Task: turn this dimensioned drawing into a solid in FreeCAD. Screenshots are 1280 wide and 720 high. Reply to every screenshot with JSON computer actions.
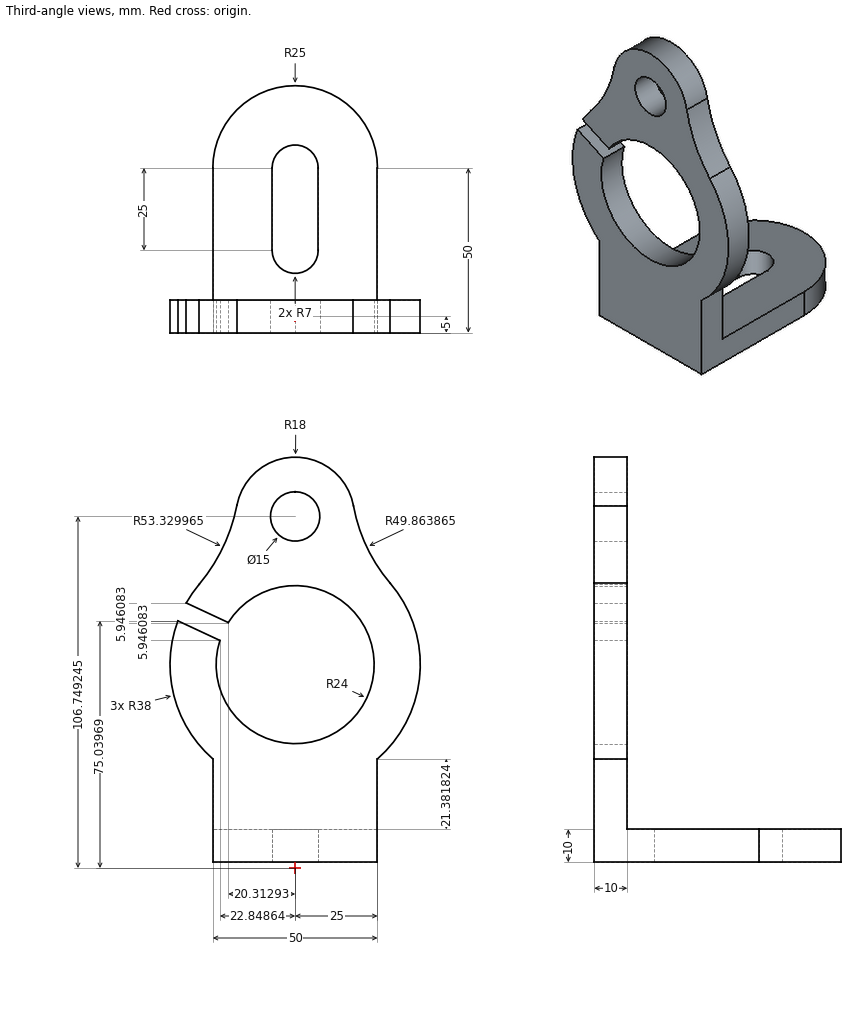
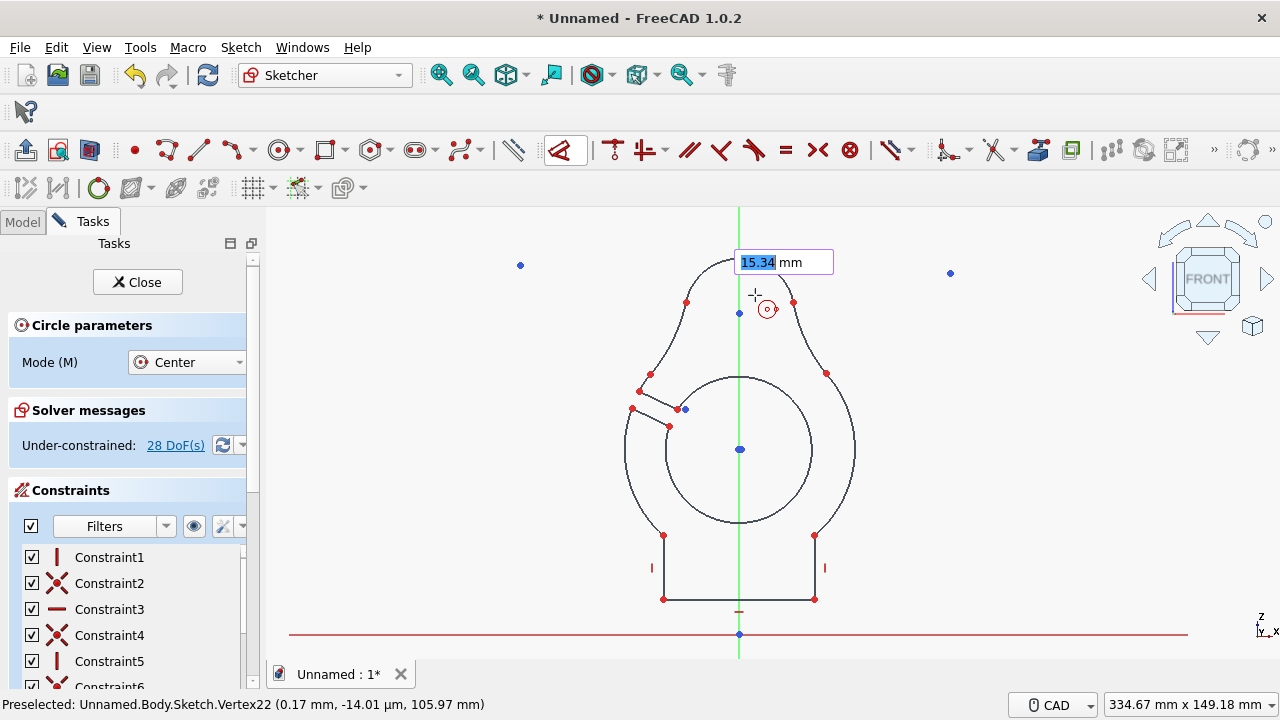
{"action": "type", "text": "15"}
{"action": "key", "text": "Return"}
{"action": "key", "text": "Escape"}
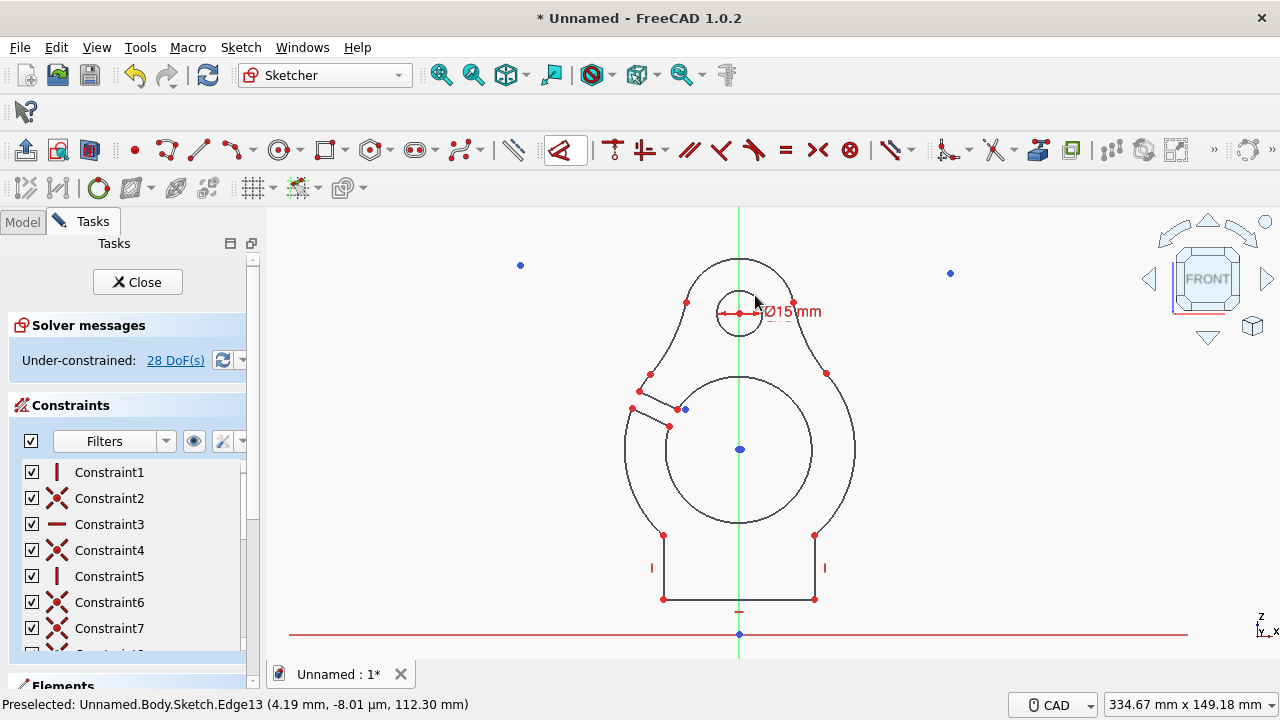
{"action": "scroll", "coordinate": [644, 383], "scroll_direction": "up", "scroll_amount": 2}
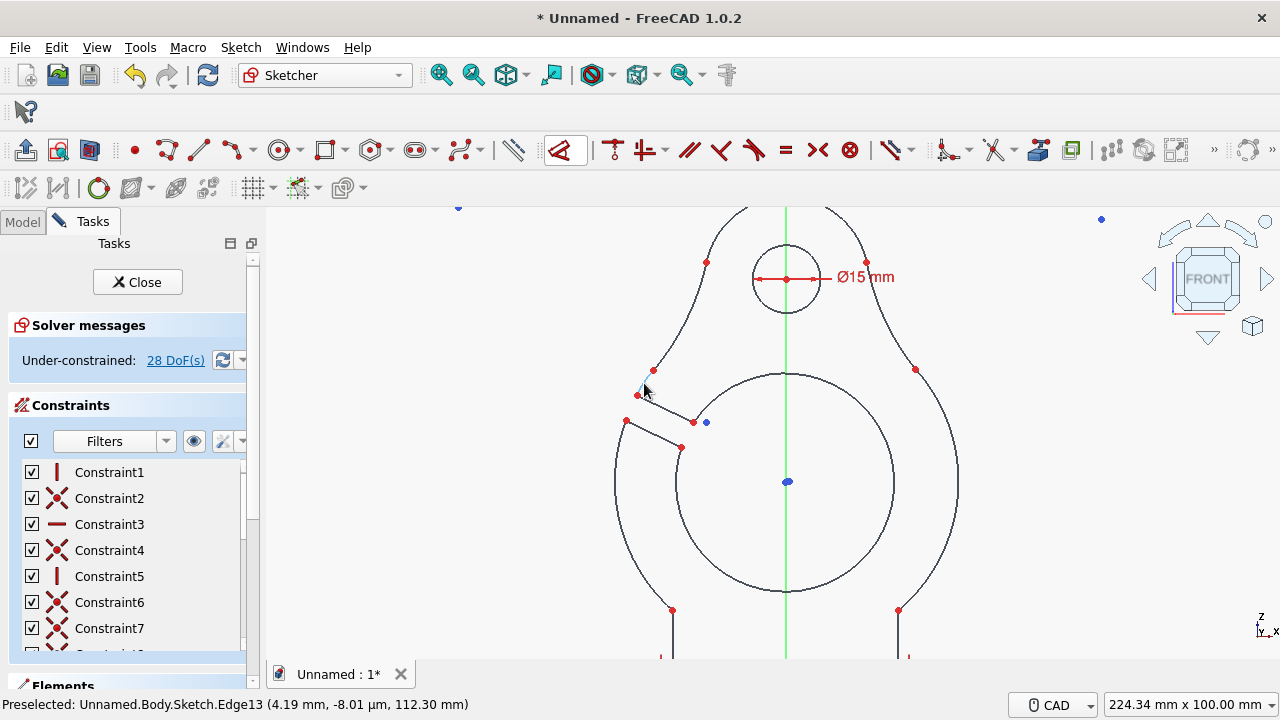
{"action": "left_click", "coordinate": [644, 382]}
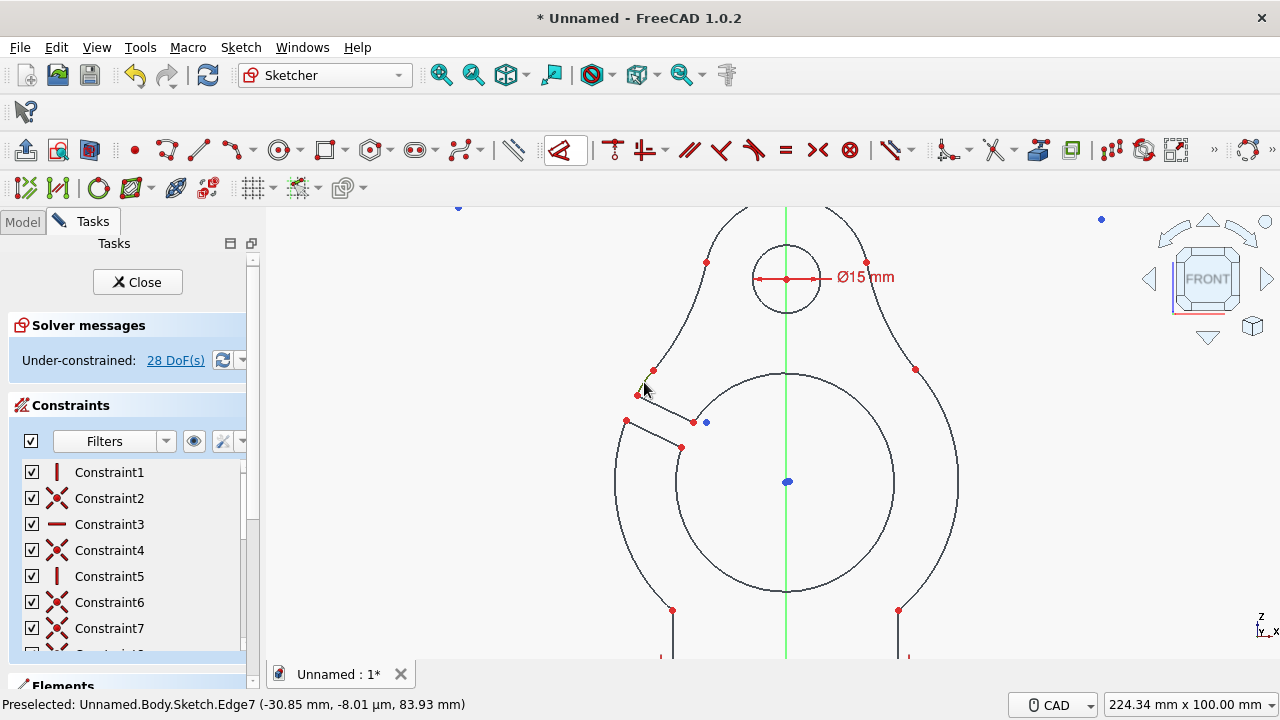
{"action": "left_click", "coordinate": [675, 341]}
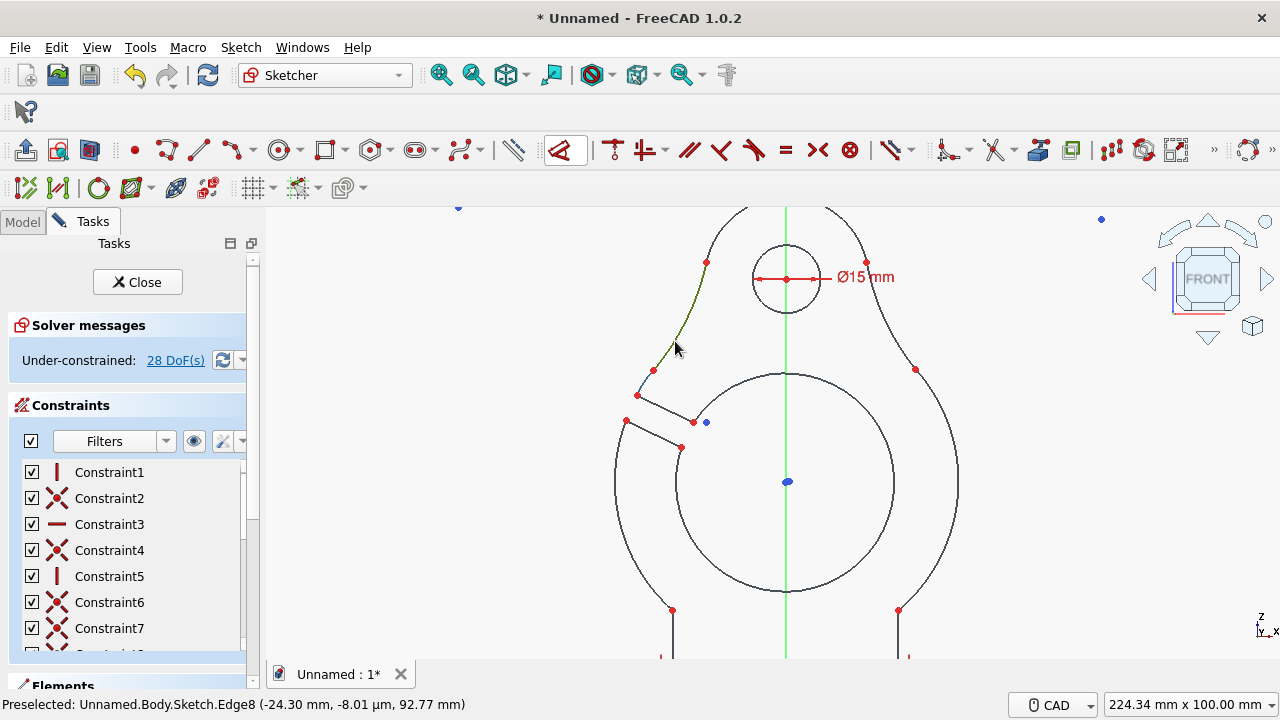
{"action": "left_click", "coordinate": [754, 150]}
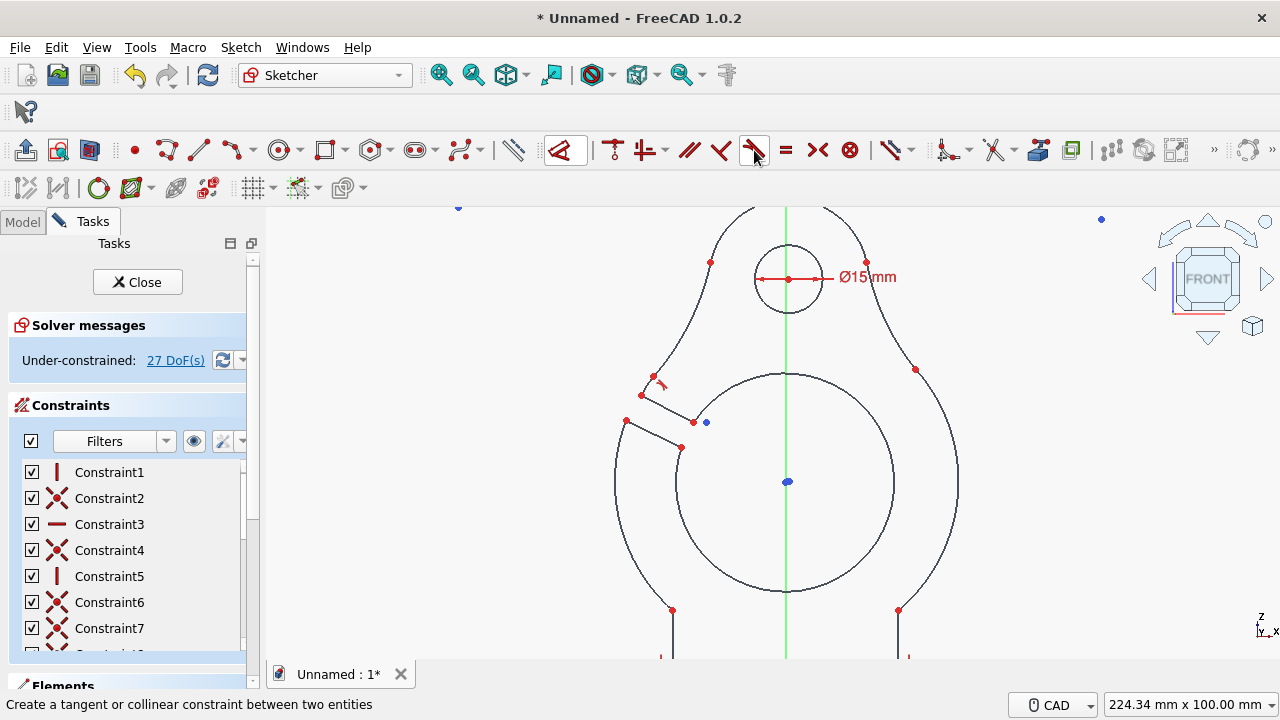
{"action": "left_click", "coordinate": [677, 346]}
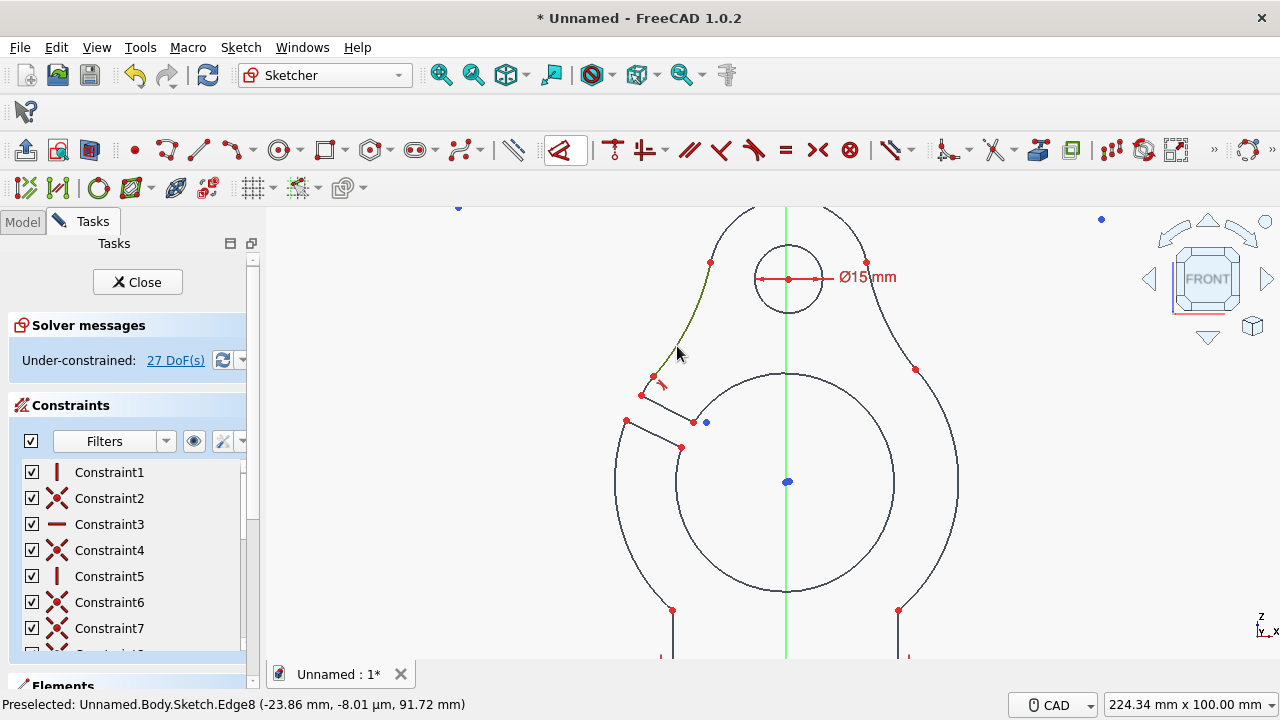
{"action": "scroll", "coordinate": [636, 398], "scroll_direction": "down", "scroll_amount": 4}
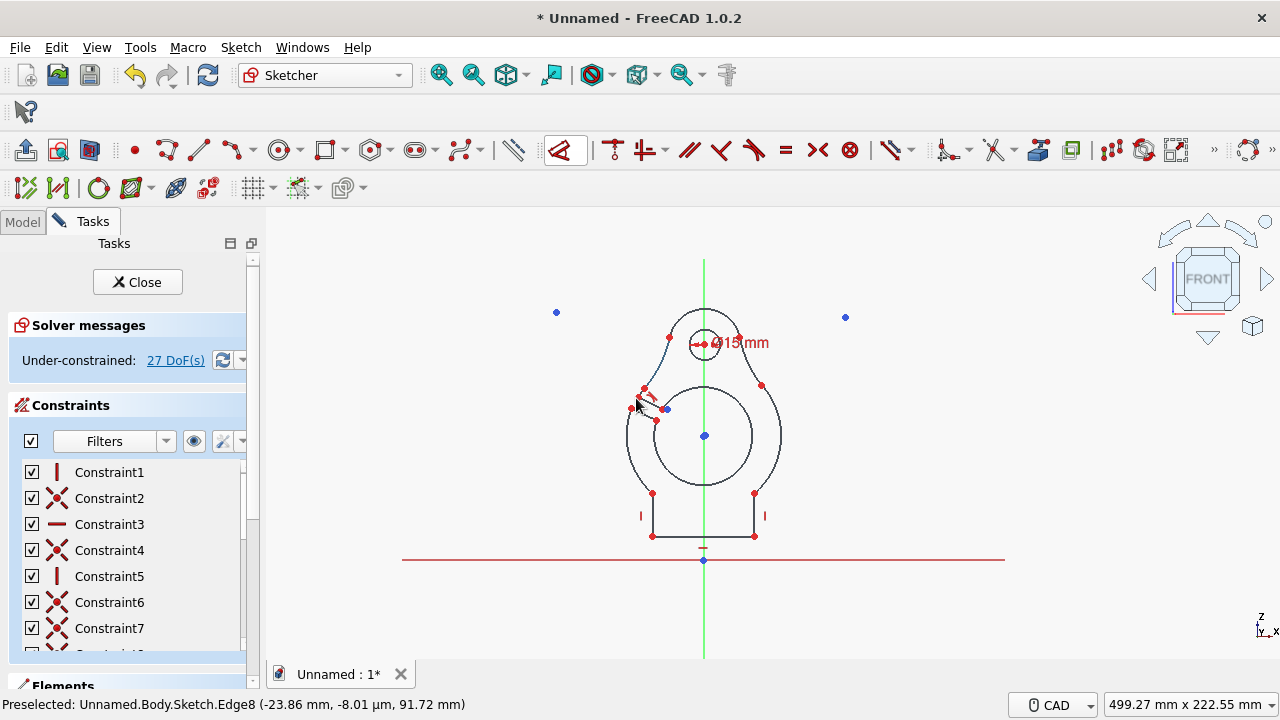
{"action": "left_click", "coordinate": [723, 314]}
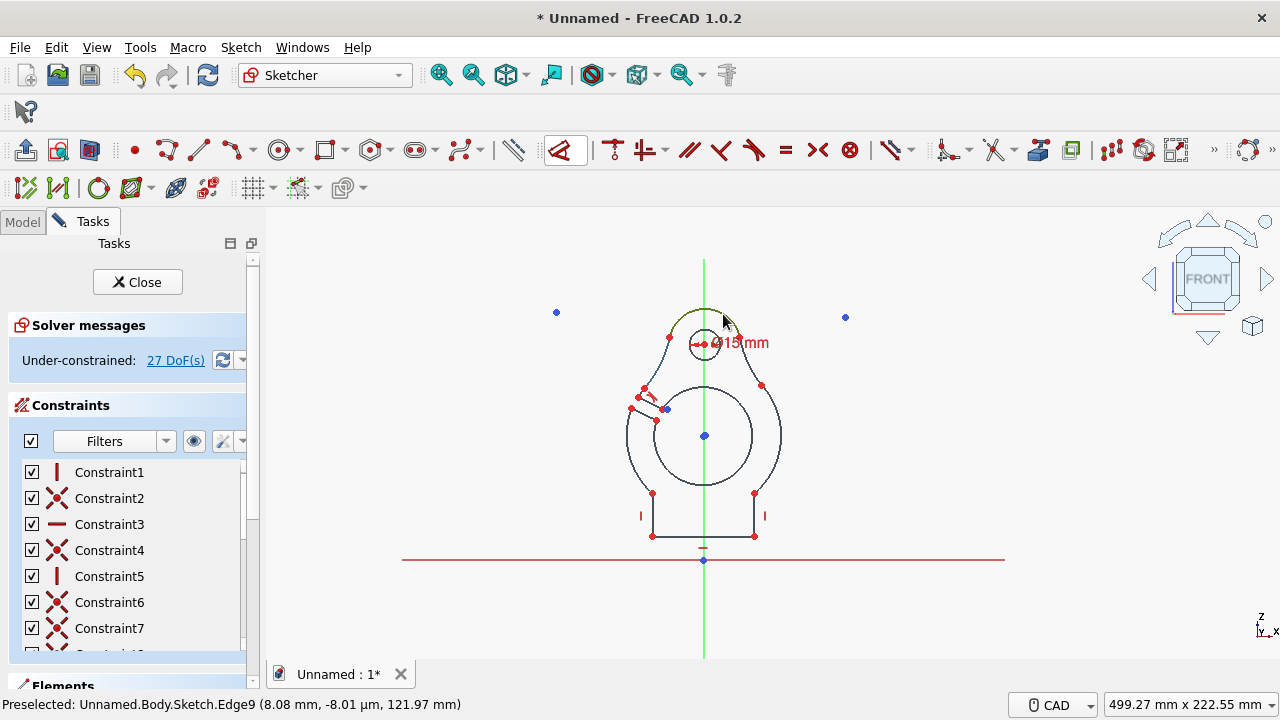
{"action": "left_click", "coordinate": [754, 150]}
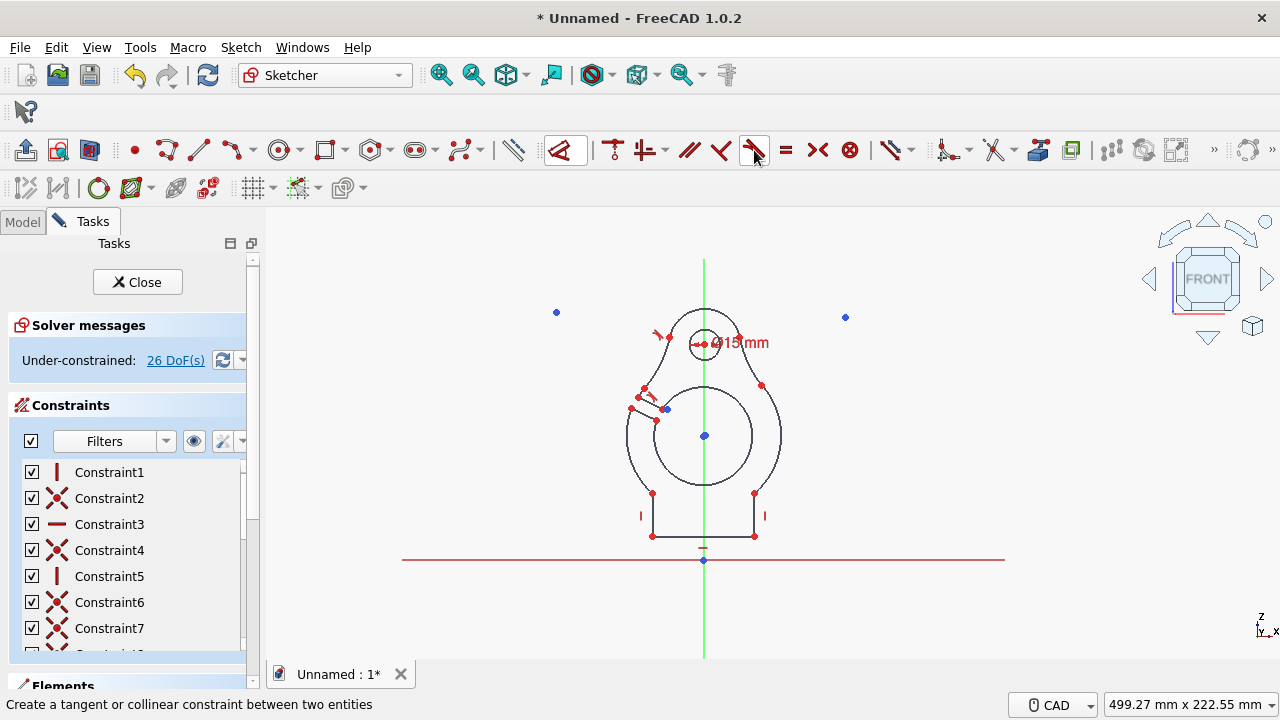
{"action": "left_click", "coordinate": [723, 314]}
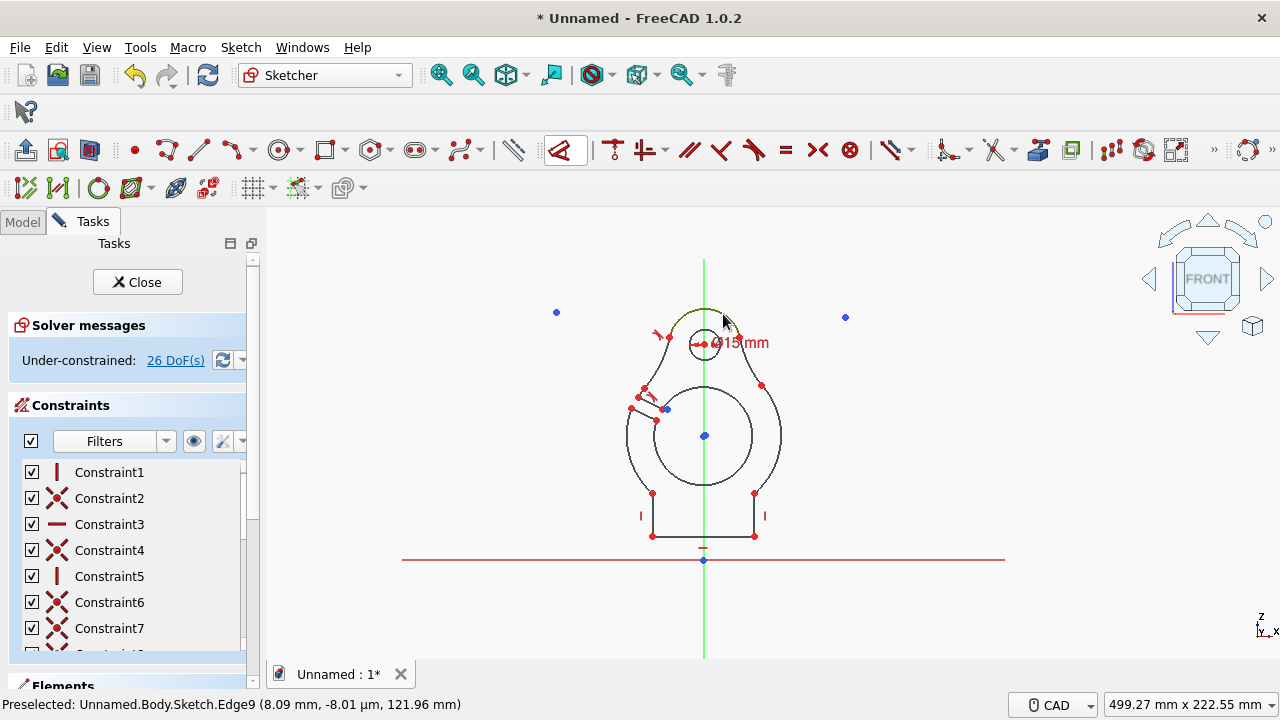
{"action": "left_click", "coordinate": [744, 353]}